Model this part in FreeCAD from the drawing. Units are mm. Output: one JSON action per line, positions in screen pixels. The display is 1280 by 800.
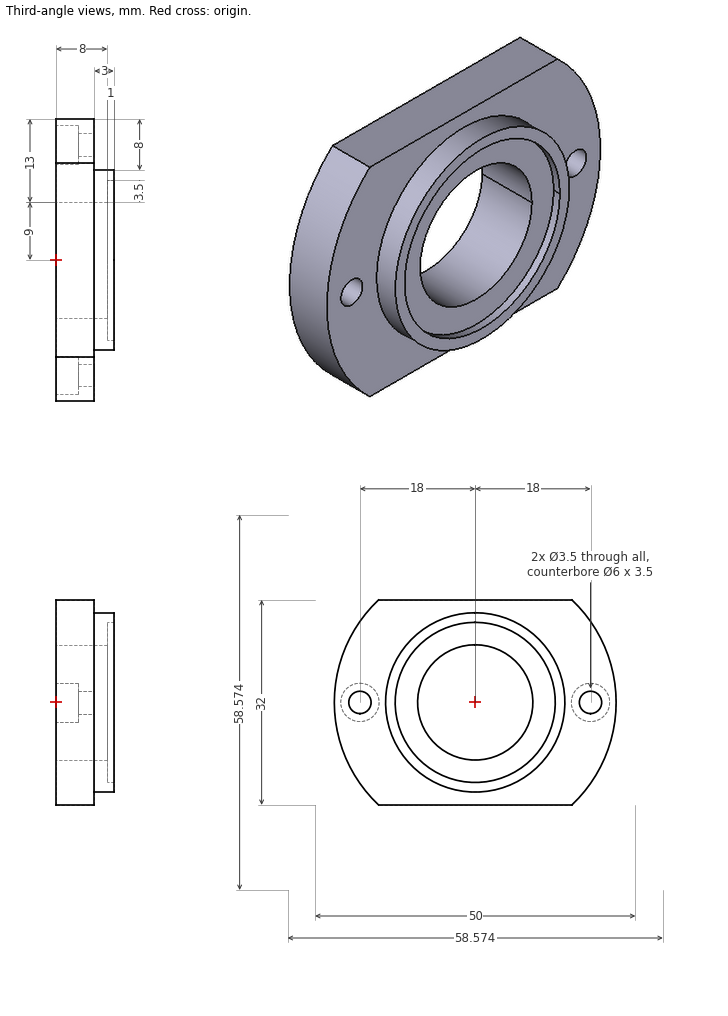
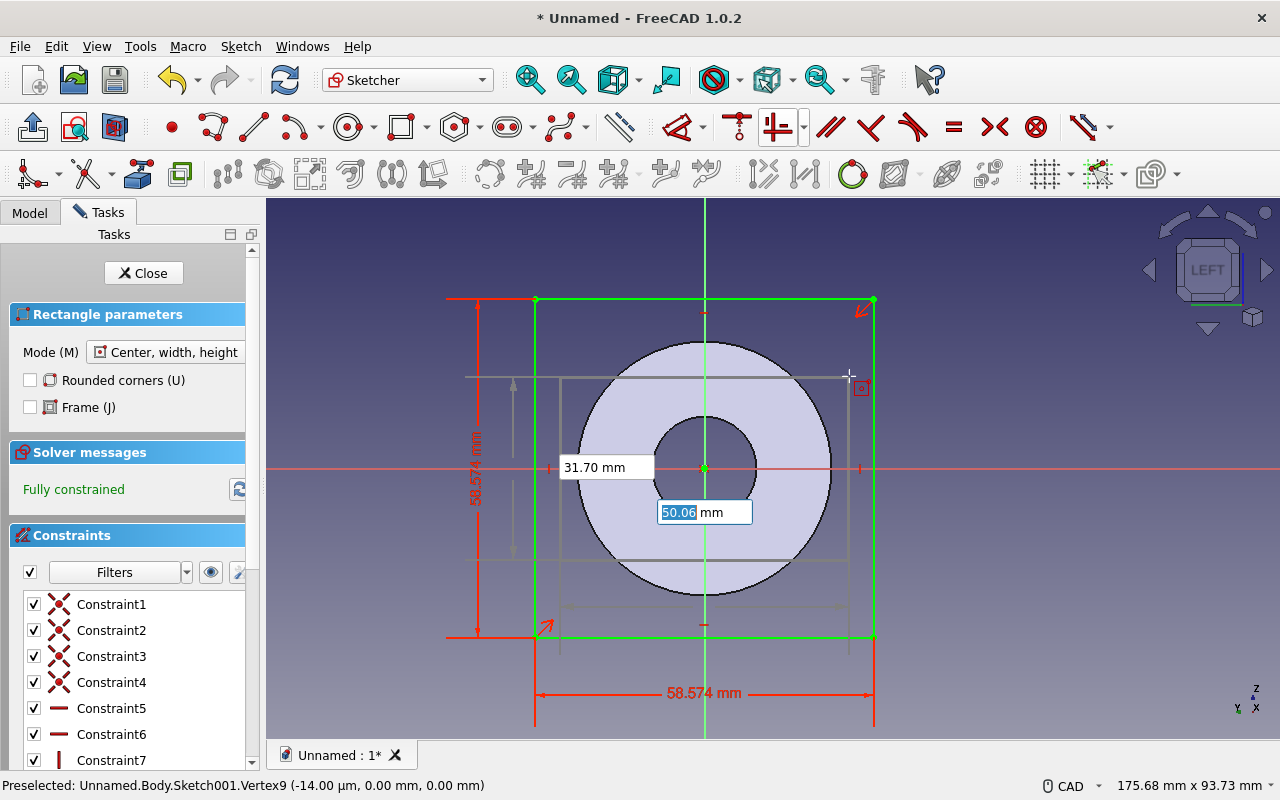
{"action": "type", "text": "50"}
{"action": "key", "text": "Tab"}
{"action": "type", "text": "32"}
{"action": "key", "text": "Return"}
{"action": "key", "text": "Escape"}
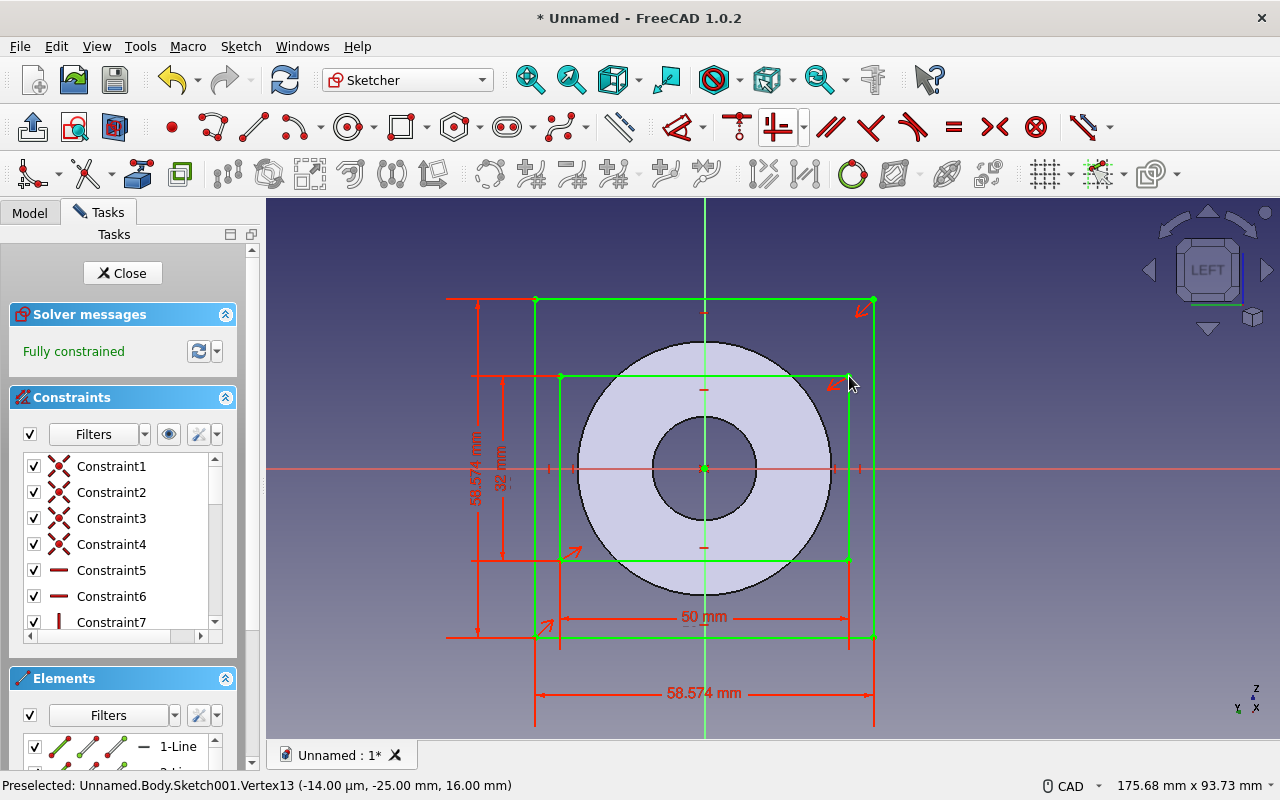
{"action": "left_click", "coordinate": [123, 273]}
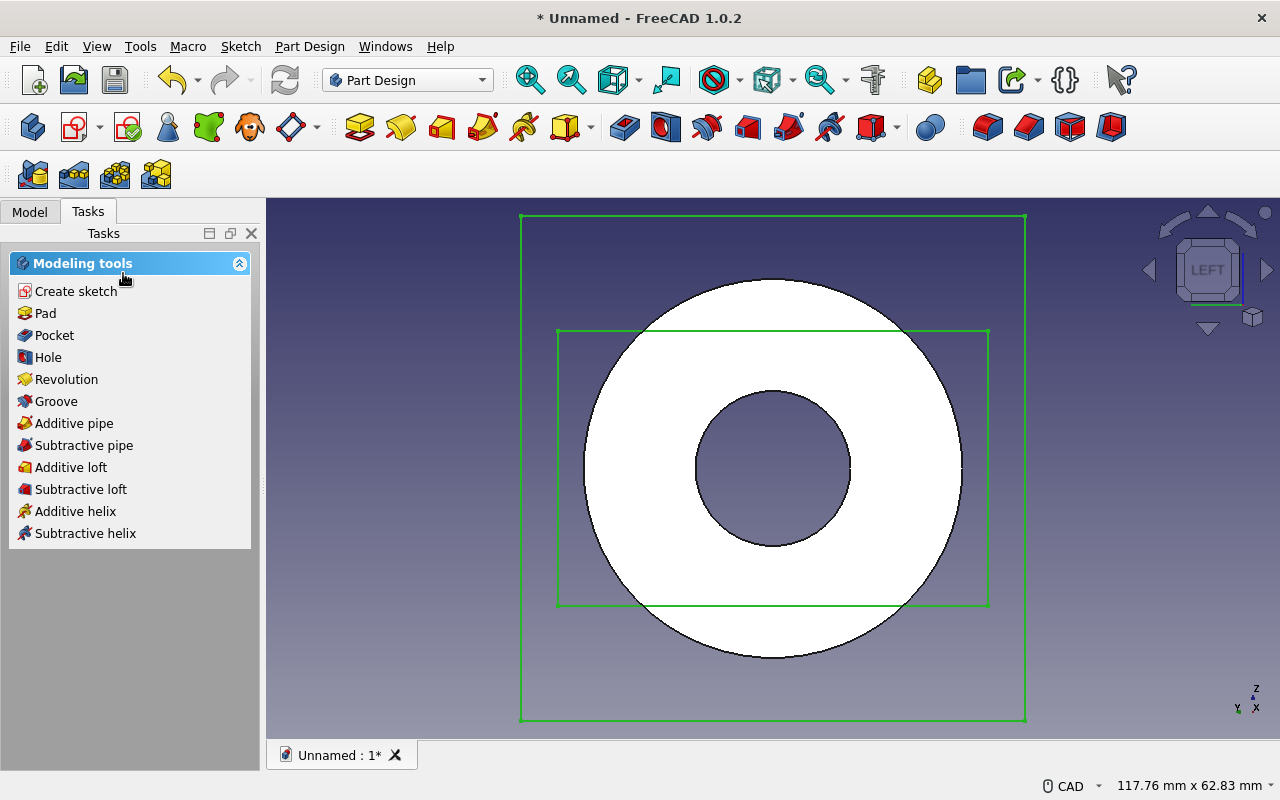
{"action": "left_click", "coordinate": [625, 128]}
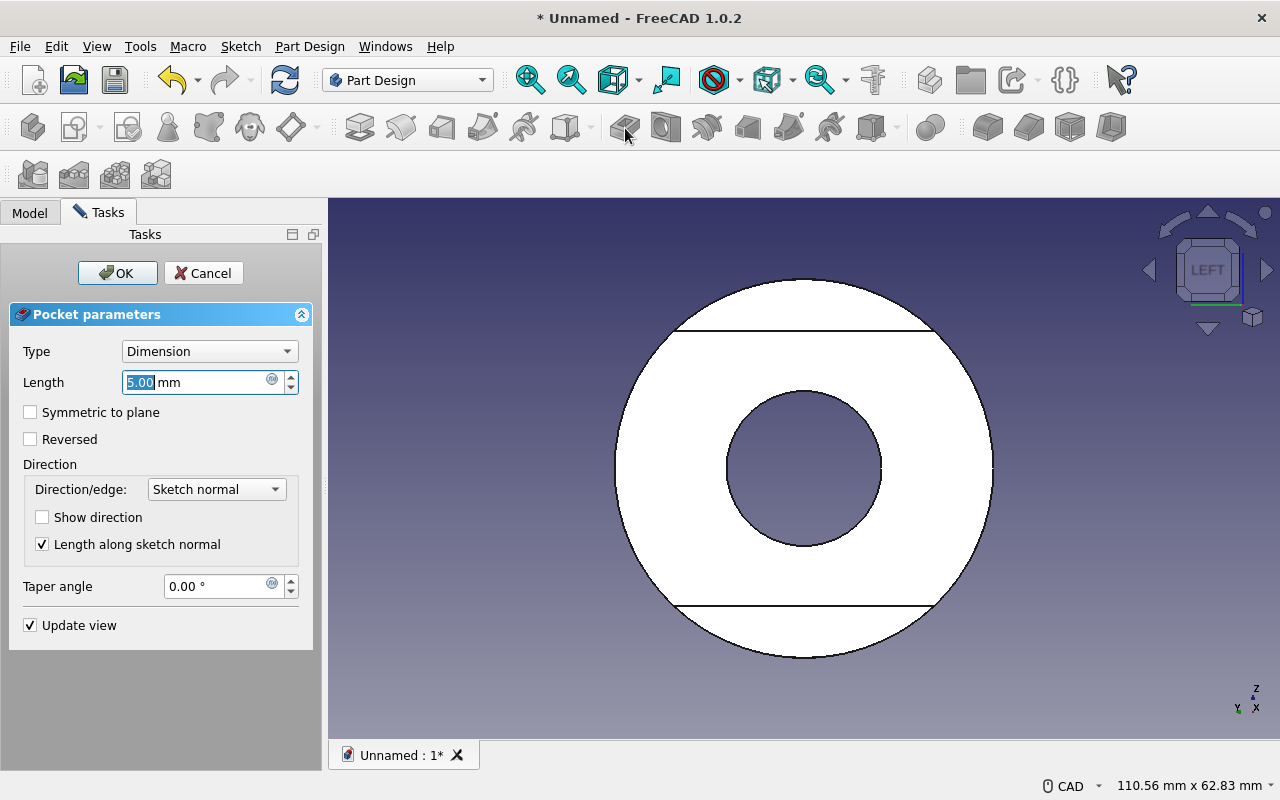
{"action": "left_click", "coordinate": [210, 352]}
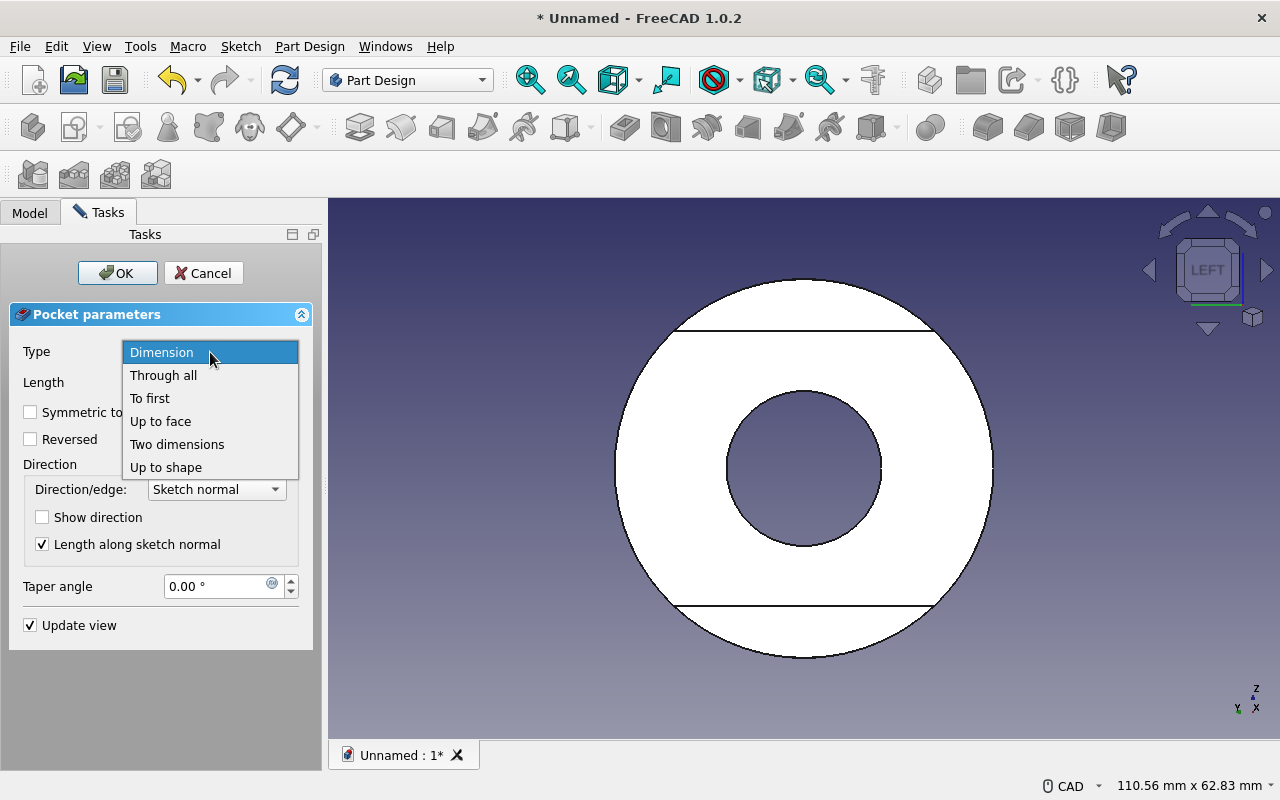
{"action": "left_click", "coordinate": [208, 376]}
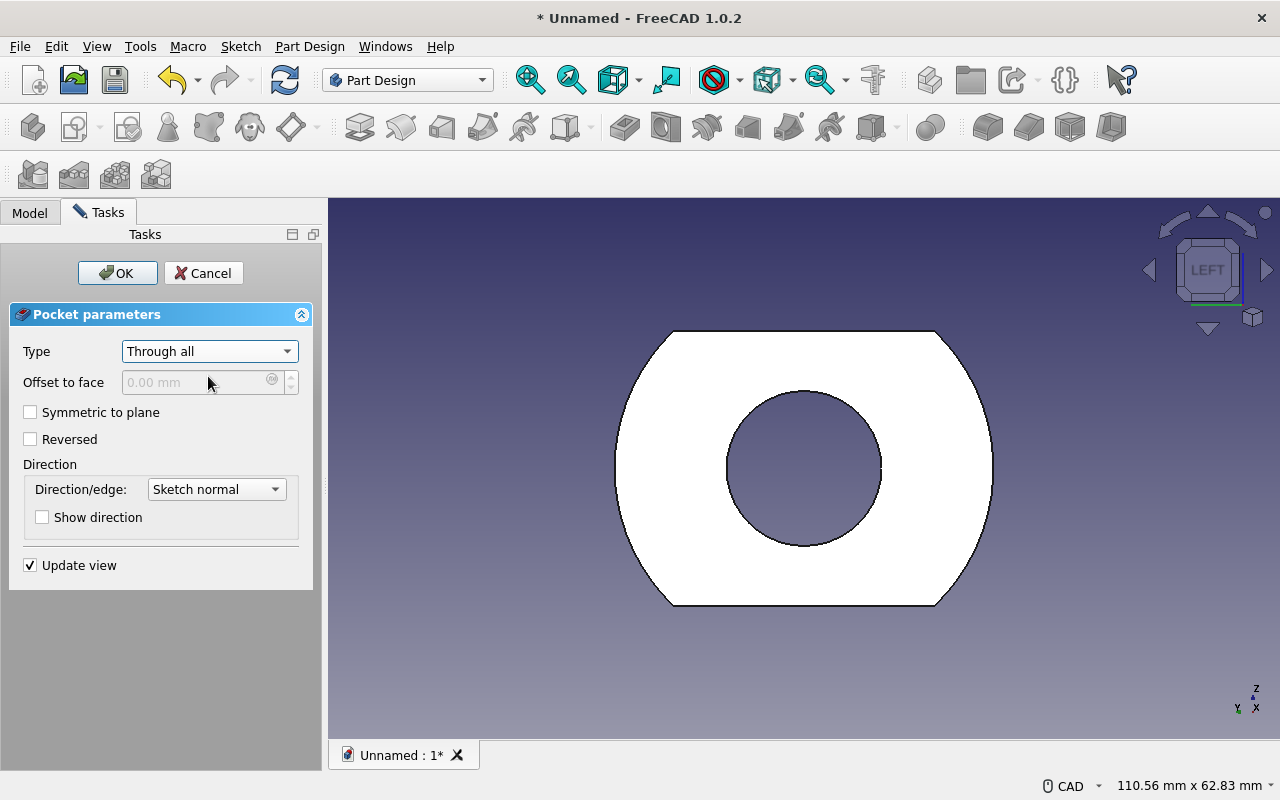
{"action": "left_click", "coordinate": [118, 273]}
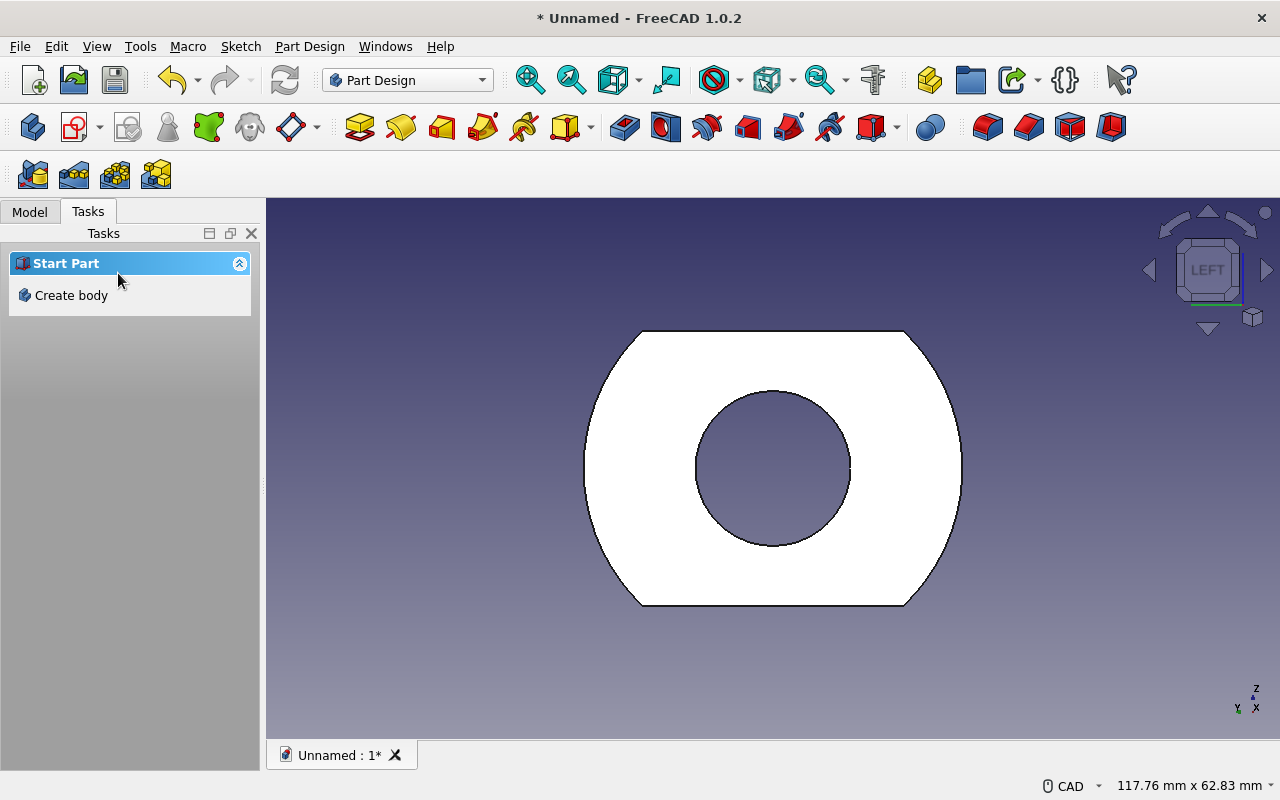
{"action": "left_click", "coordinate": [74, 128]}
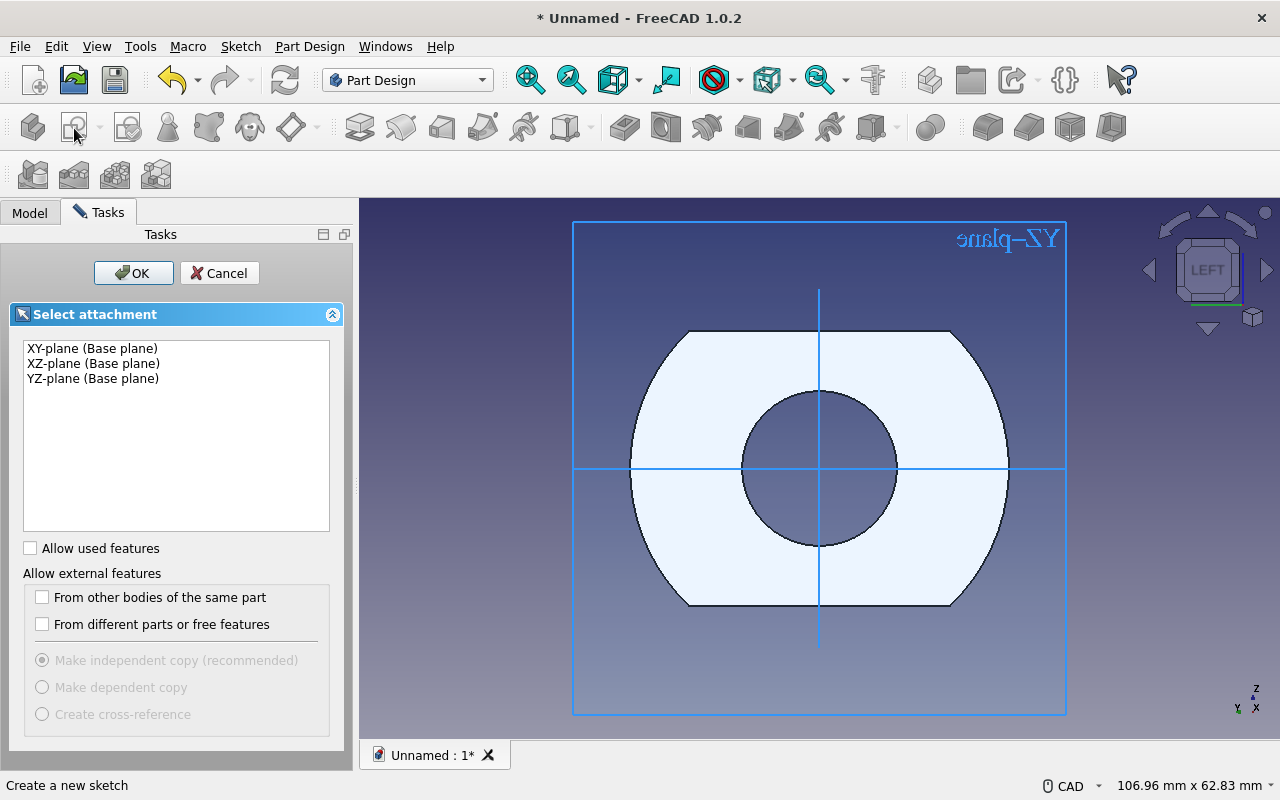
{"action": "left_click", "coordinate": [84, 378]}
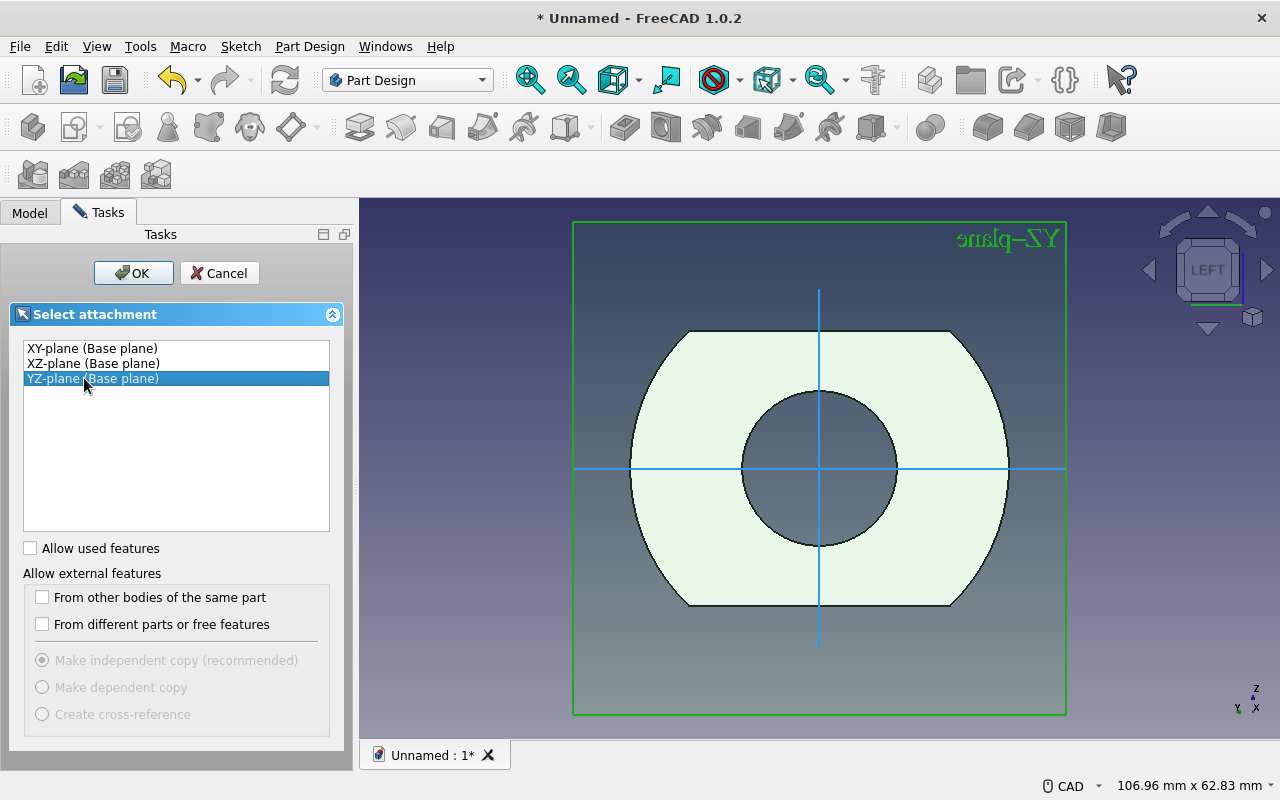
{"action": "left_click", "coordinate": [134, 273]}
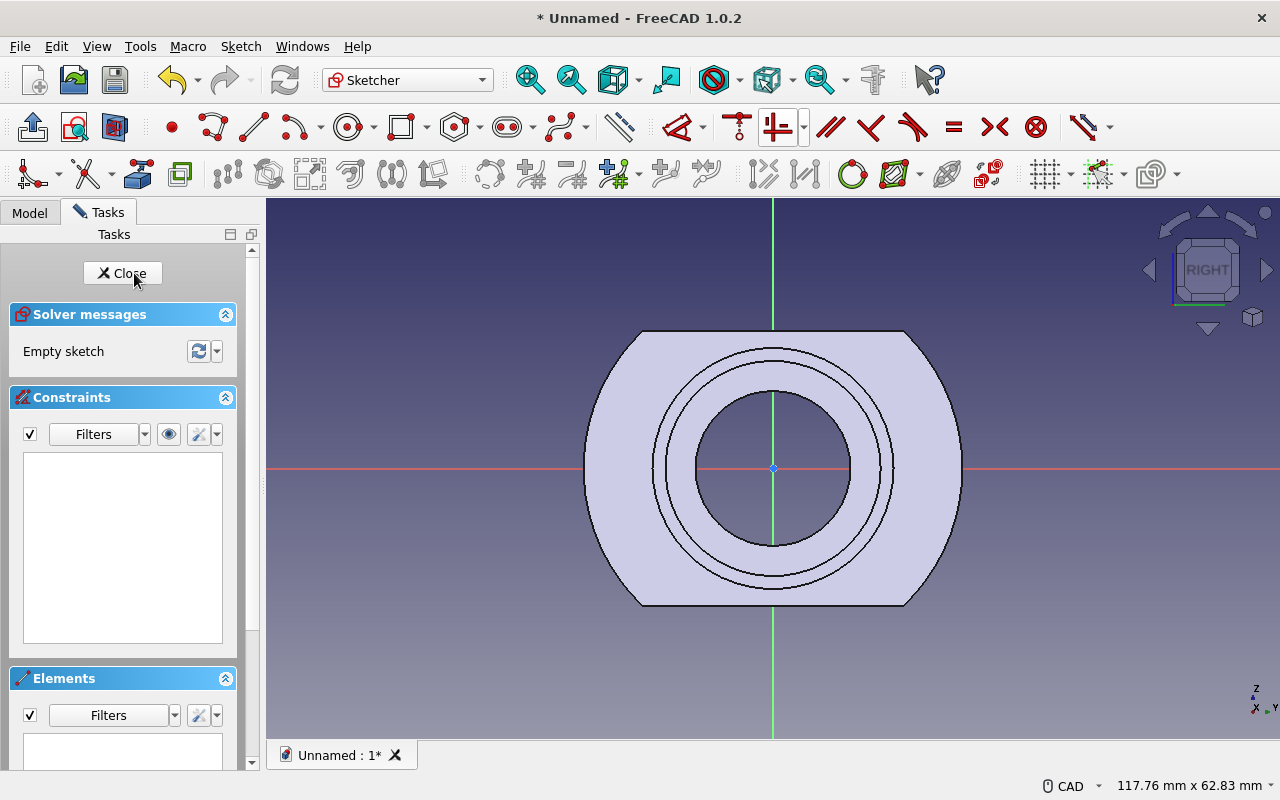
{"action": "left_click", "coordinate": [115, 128]}